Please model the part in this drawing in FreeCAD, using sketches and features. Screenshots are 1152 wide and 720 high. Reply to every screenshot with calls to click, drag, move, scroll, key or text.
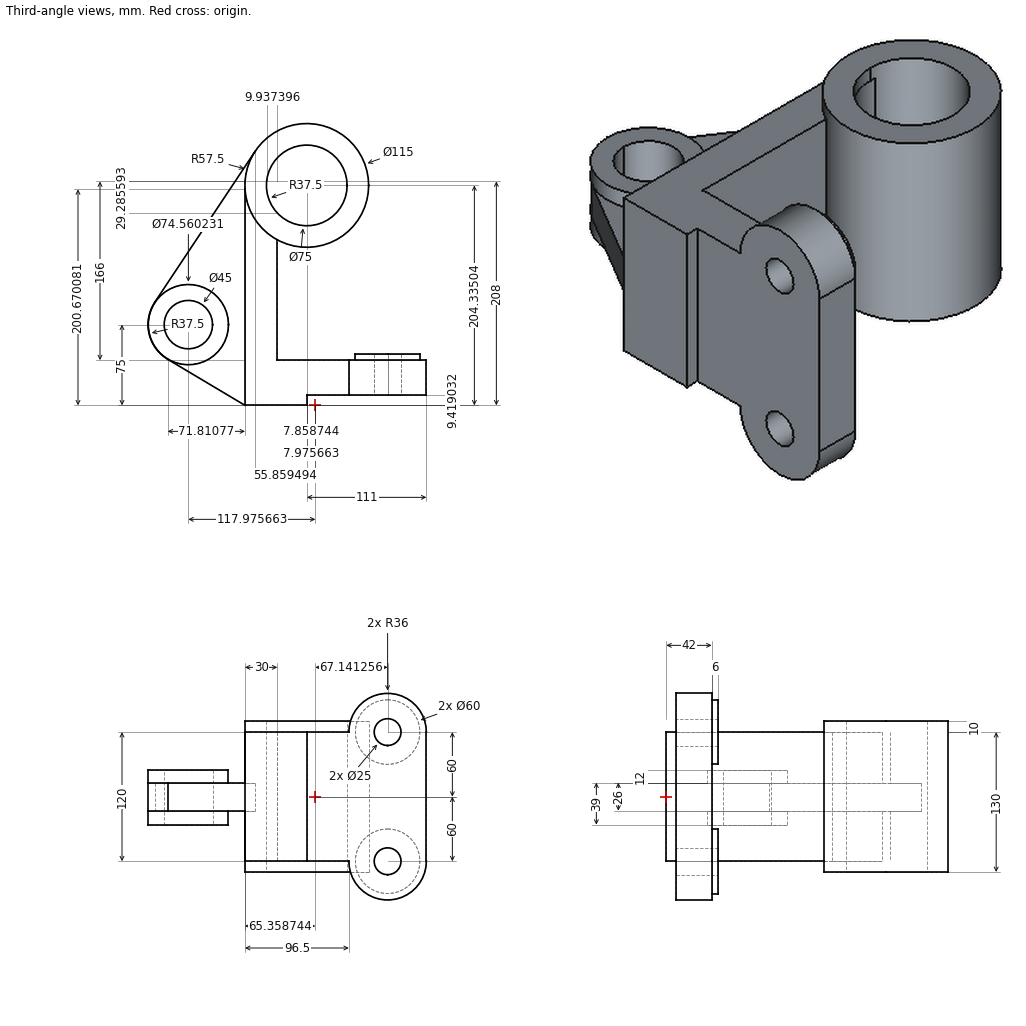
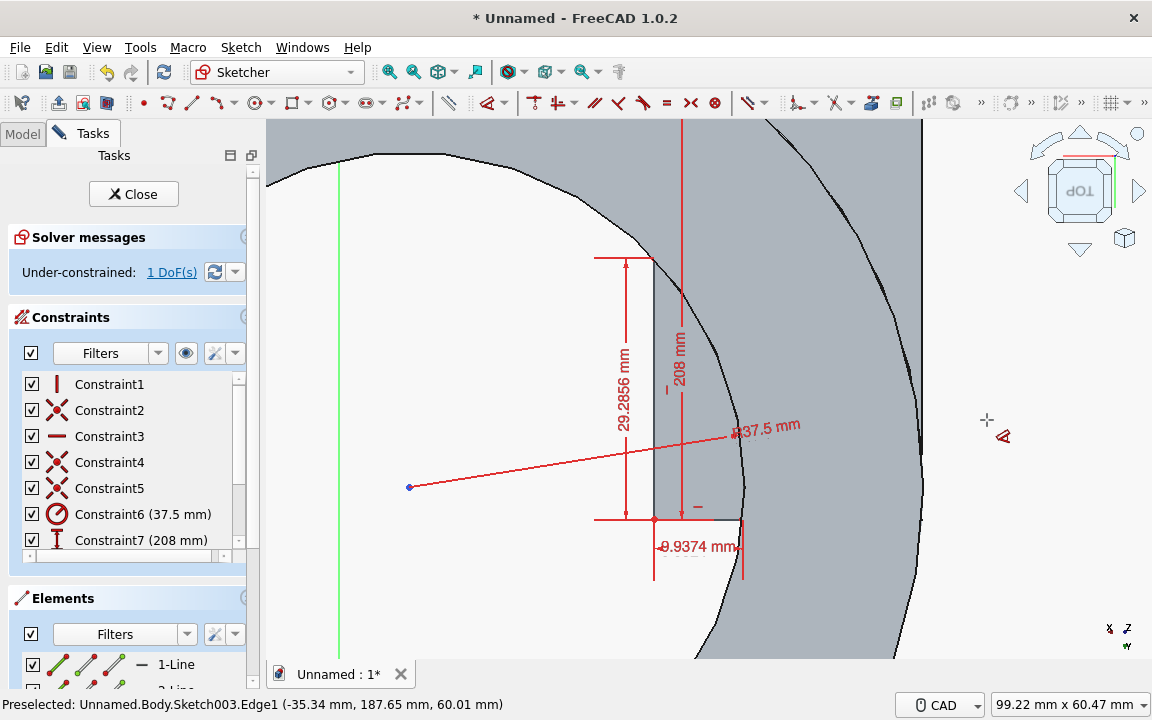
click(410, 487)
click(374, 521)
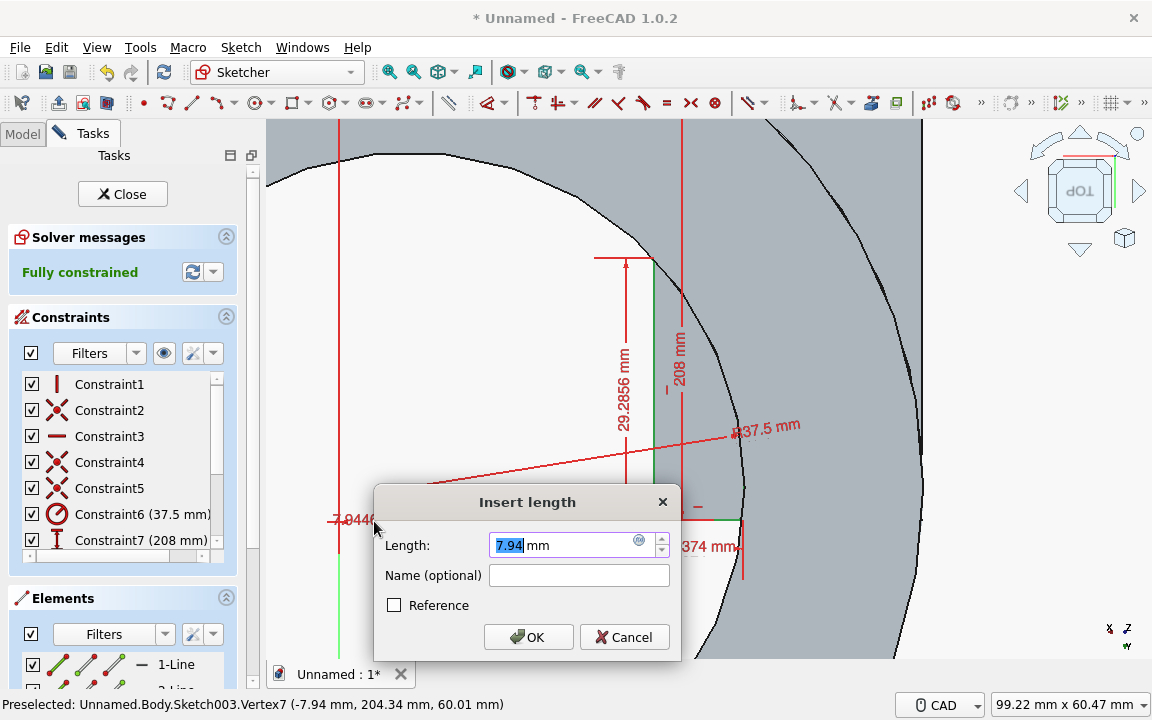
text(7.975663)
key(Return)
key(Escape)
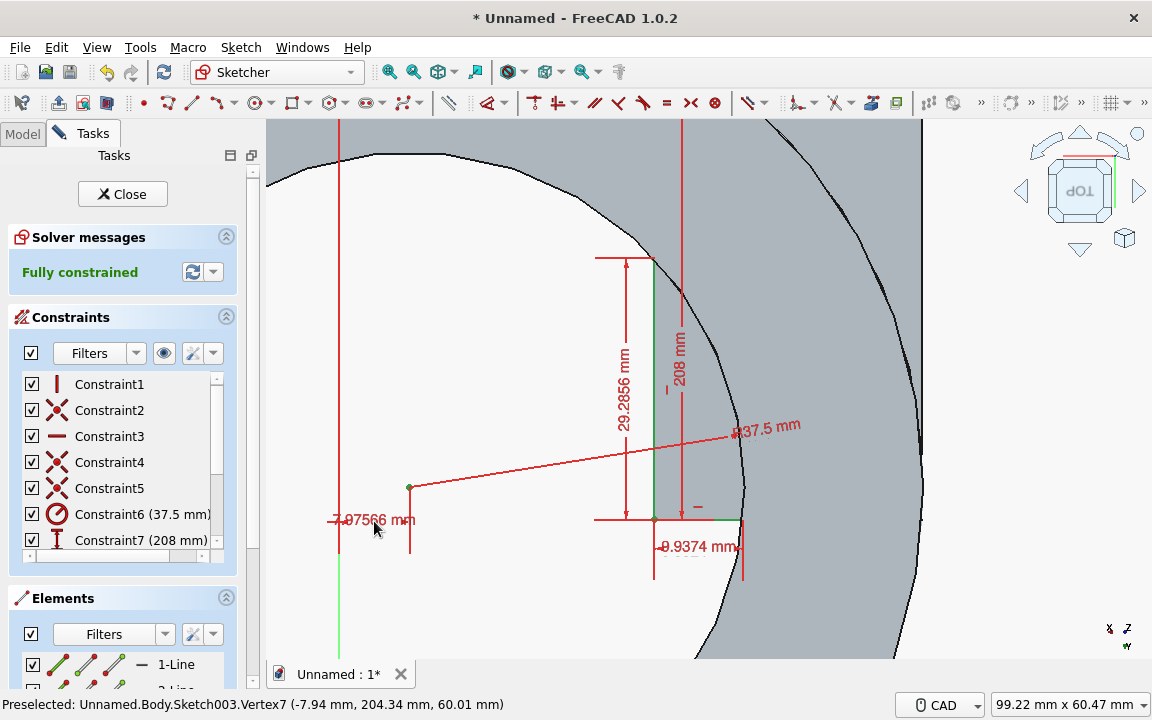
click(123, 194)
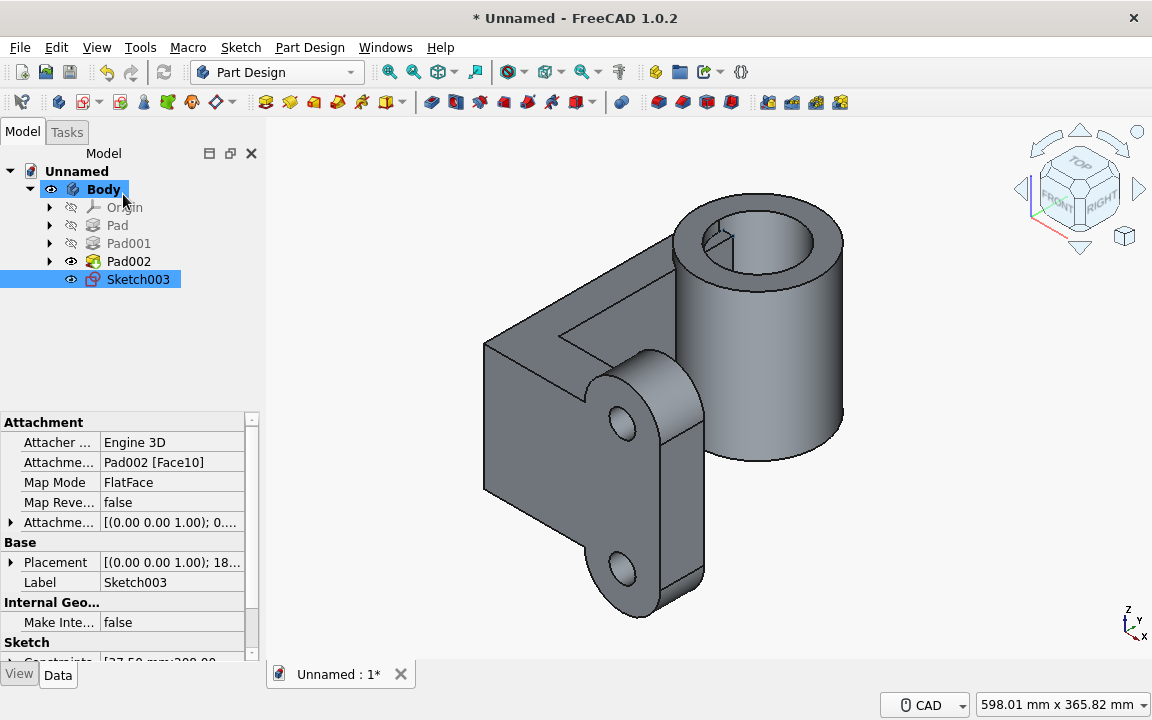
click(432, 102)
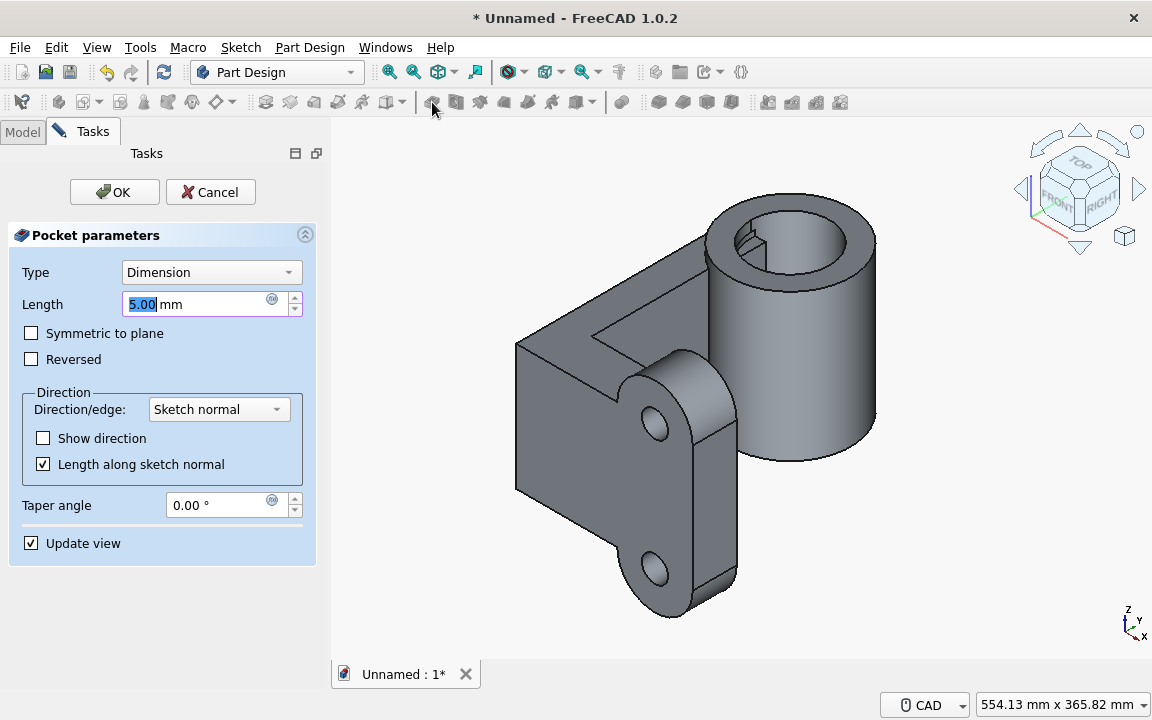
text(130)
key(Tab)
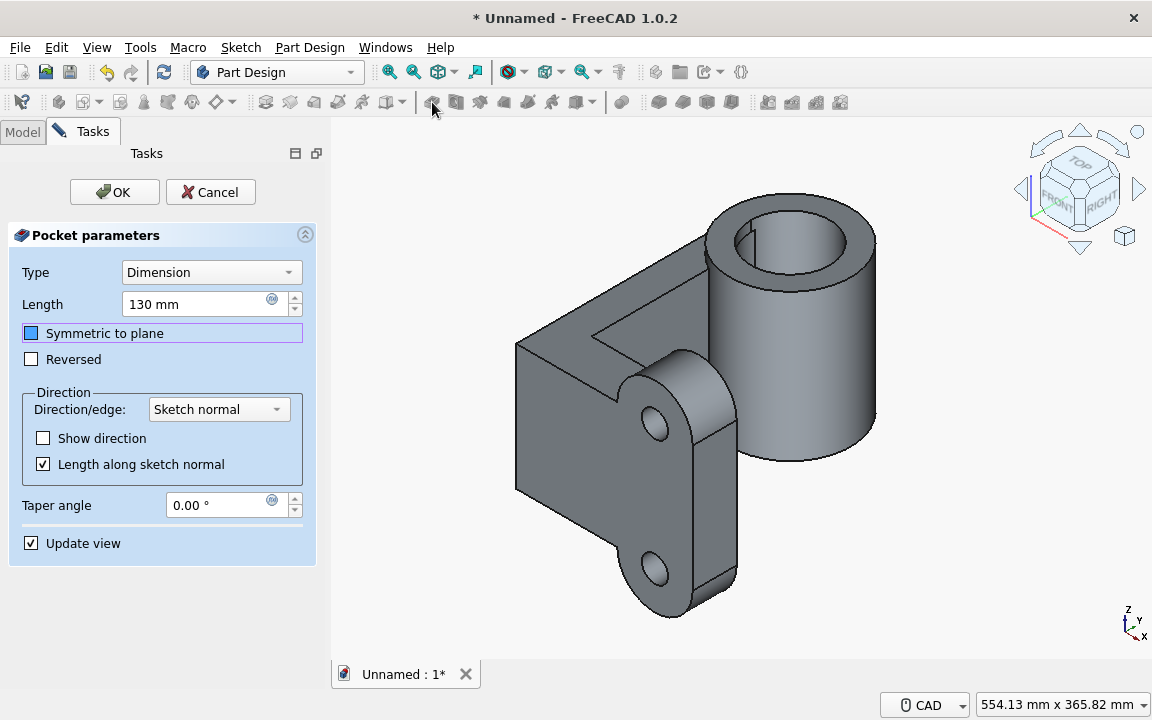
click(115, 192)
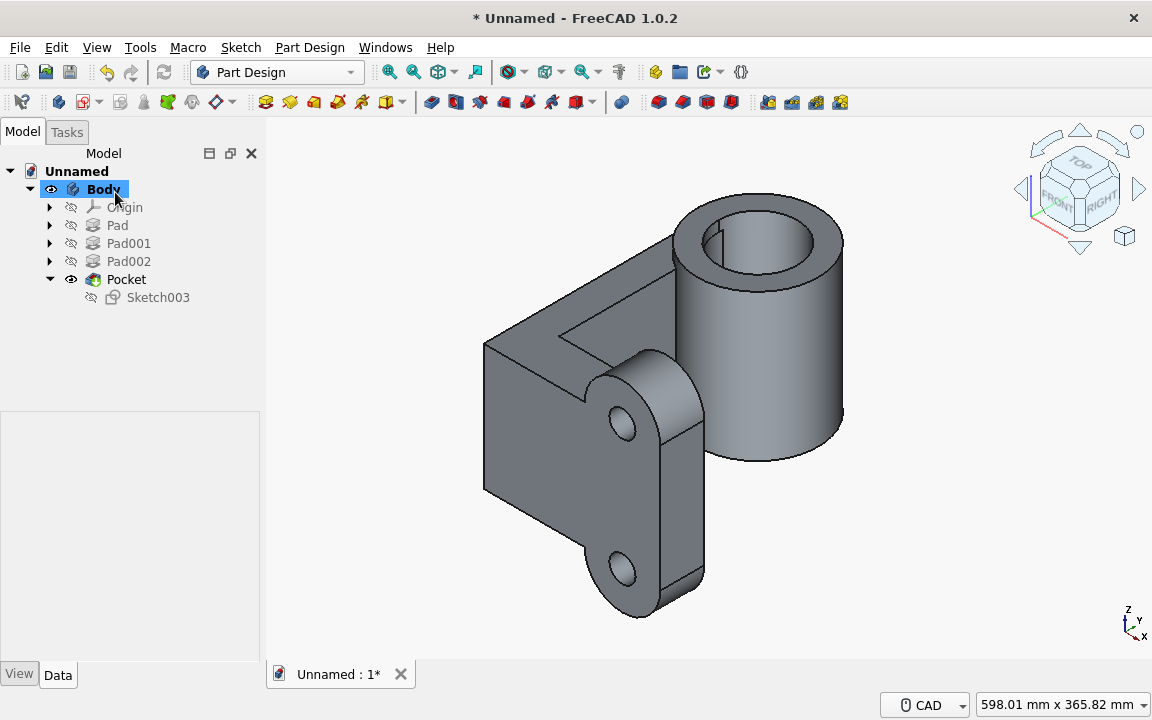
click(84, 102)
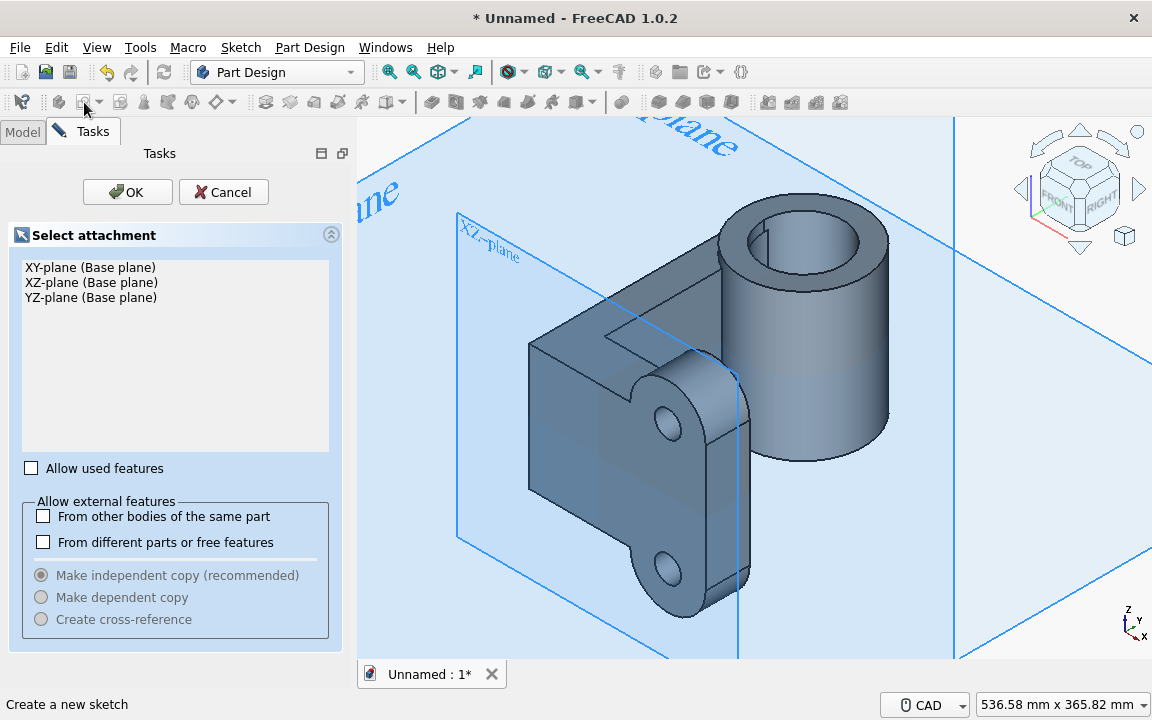
click(82, 268)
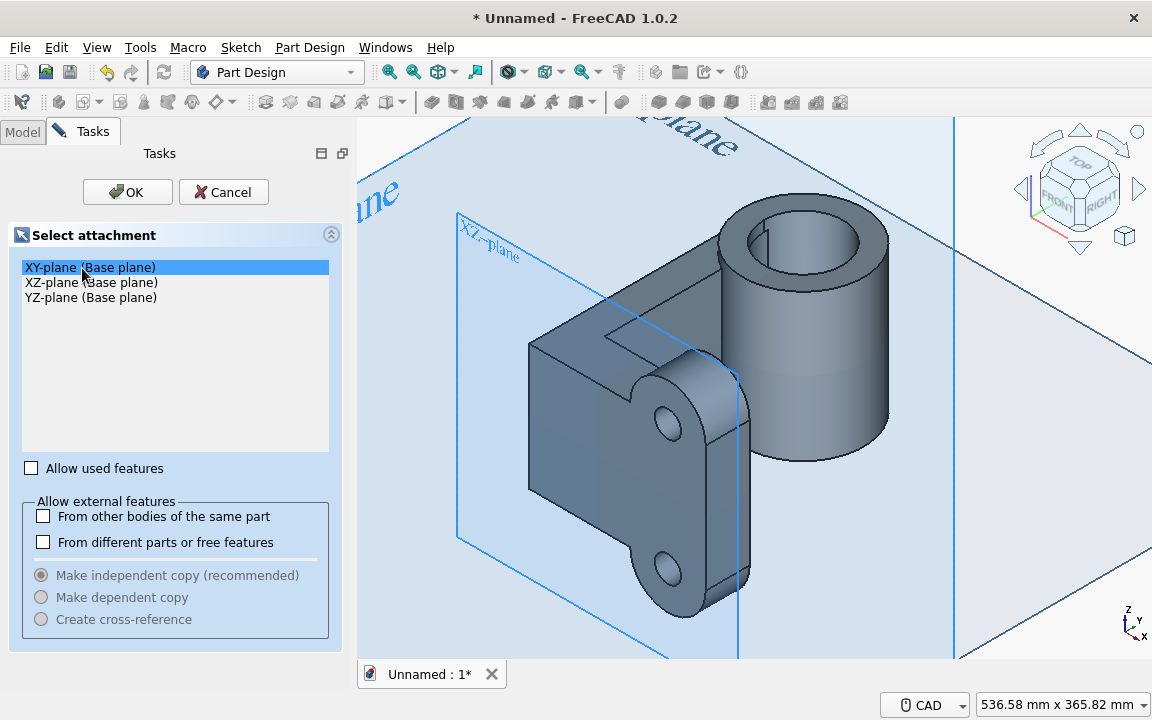
click(128, 192)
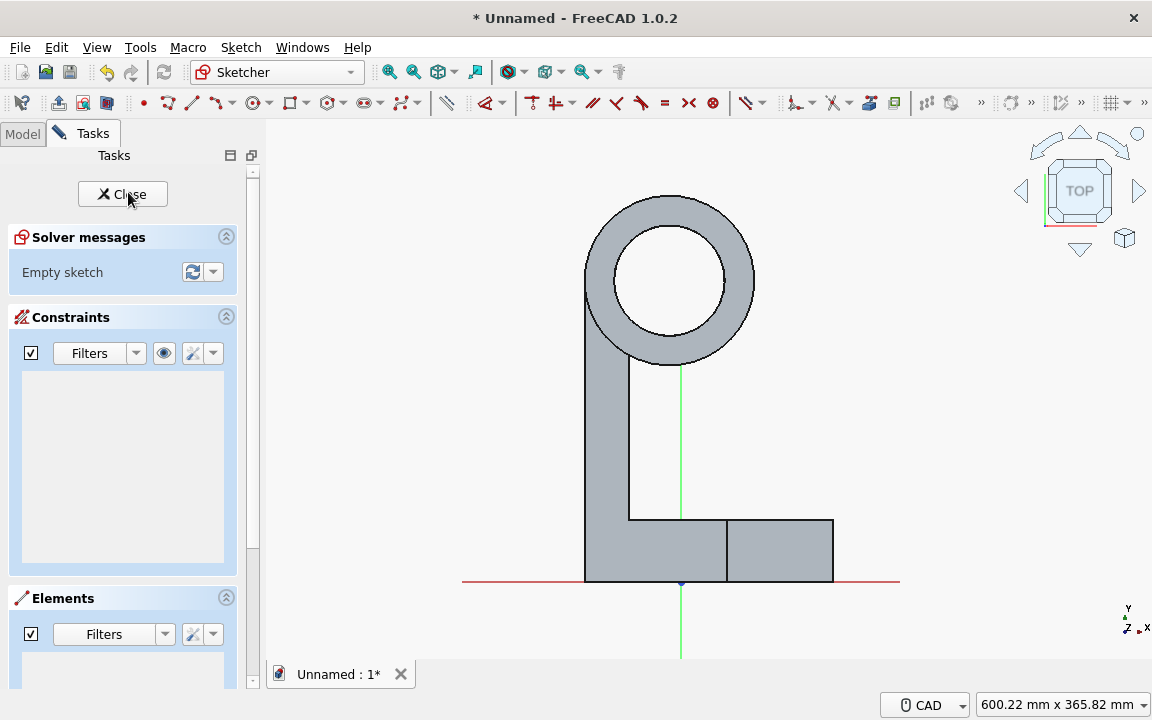
click(108, 104)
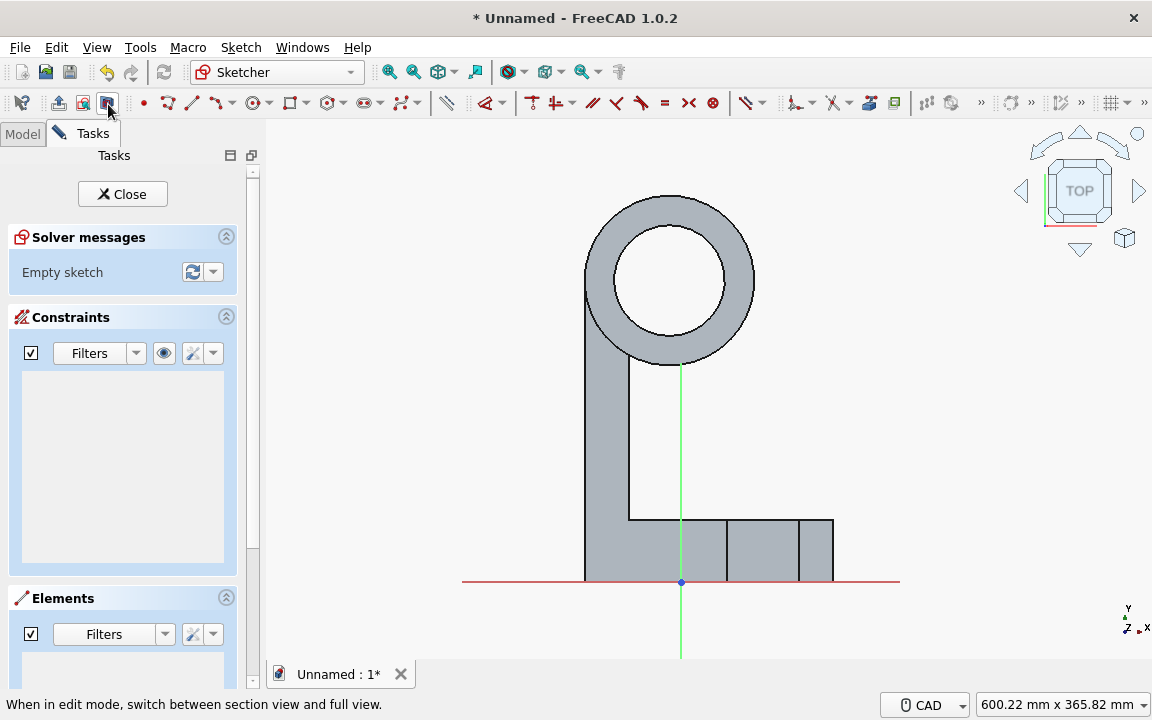
click(168, 104)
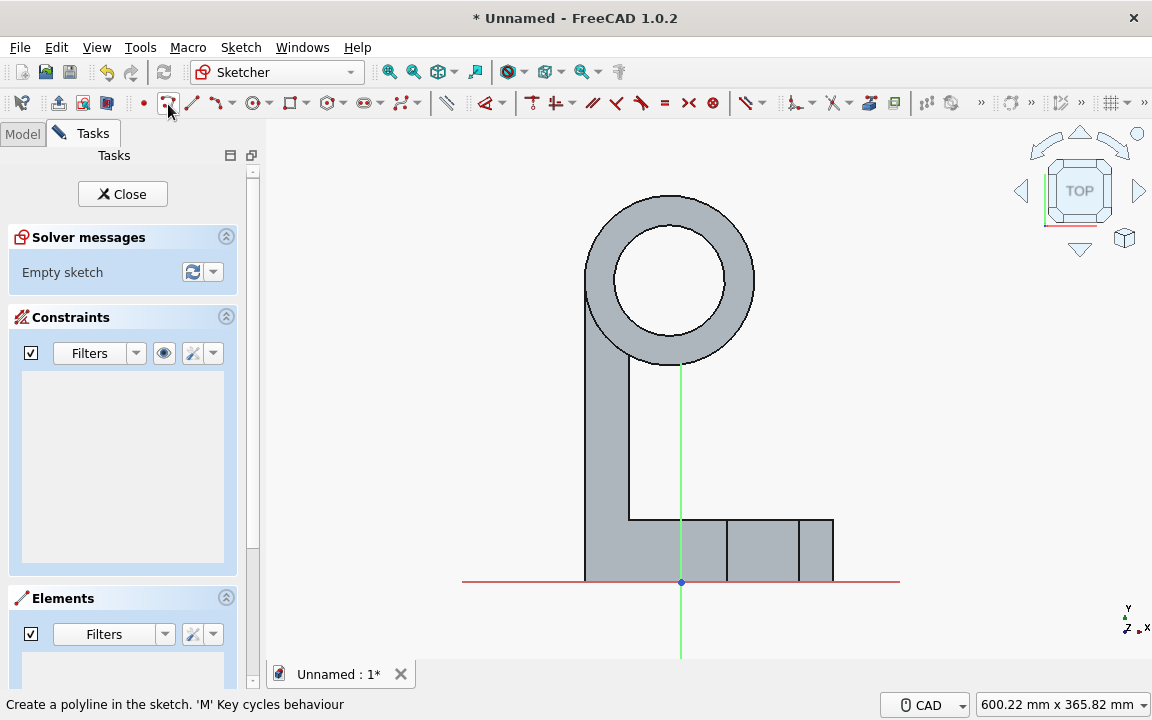
click(479, 519)
click(585, 582)
click(585, 286)
right_click(585, 286)